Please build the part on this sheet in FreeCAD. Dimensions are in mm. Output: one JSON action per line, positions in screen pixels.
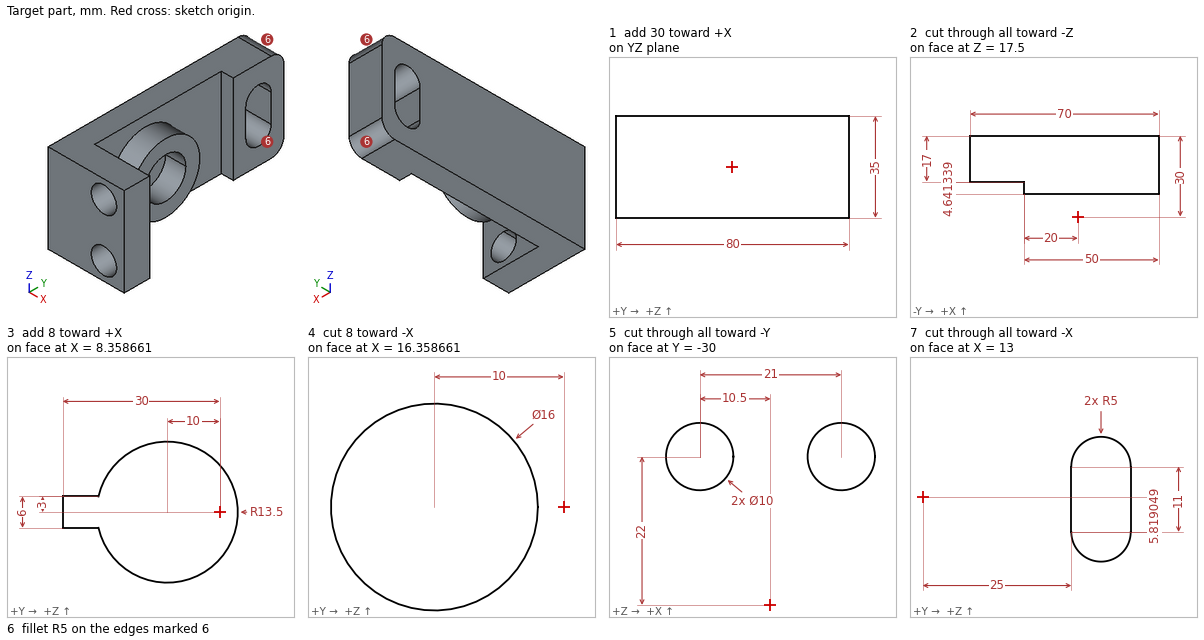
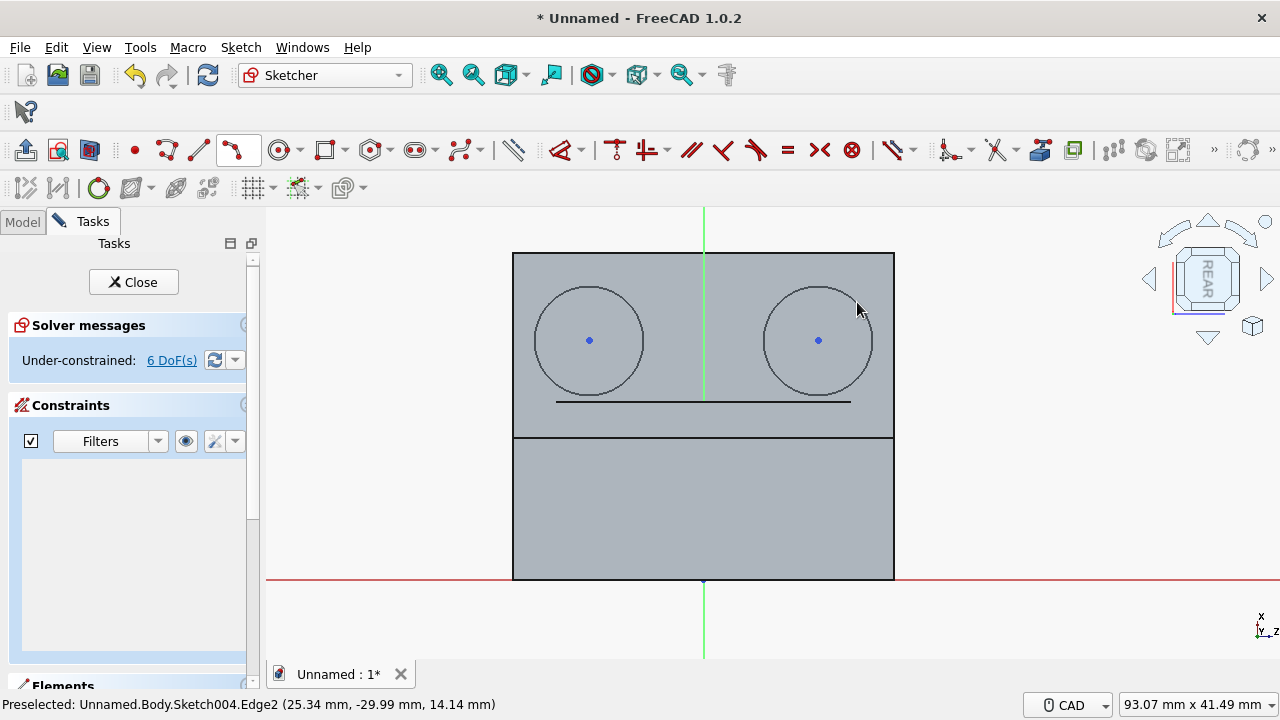
{"action": "left_click", "coordinate": [627, 302]}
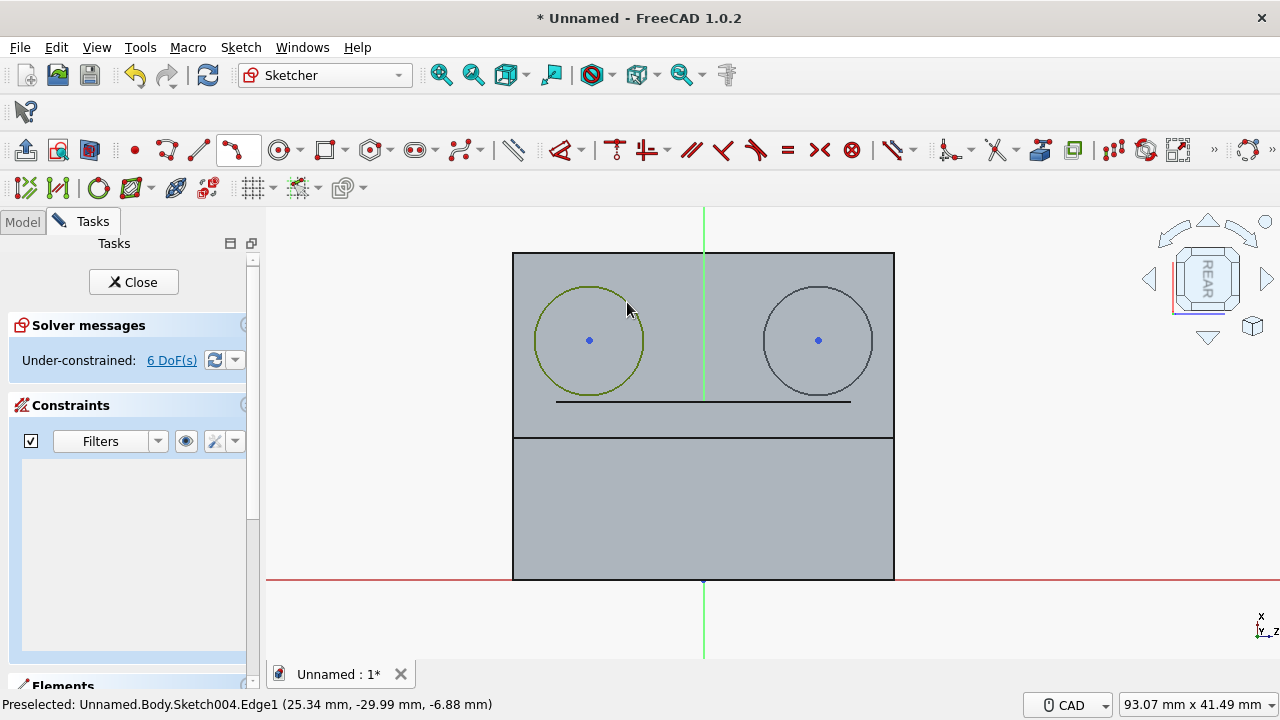
{"action": "left_click", "coordinate": [856, 302]}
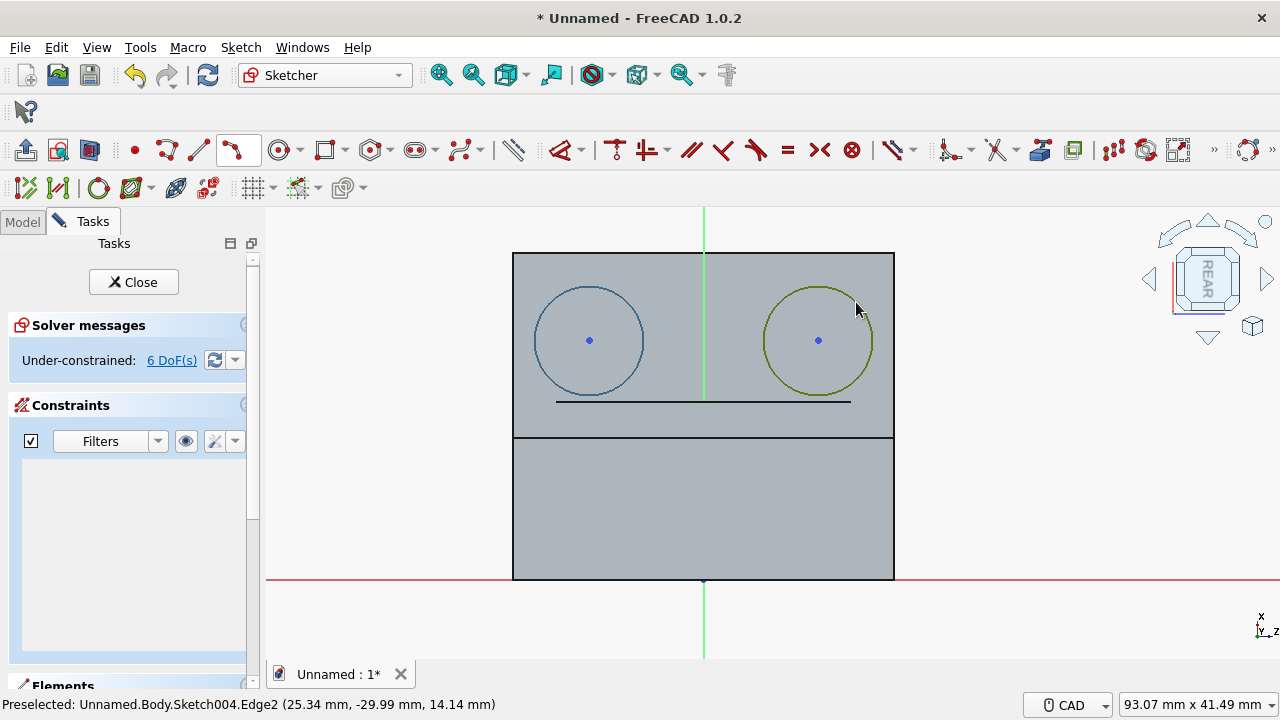
{"action": "left_click", "coordinate": [788, 150]}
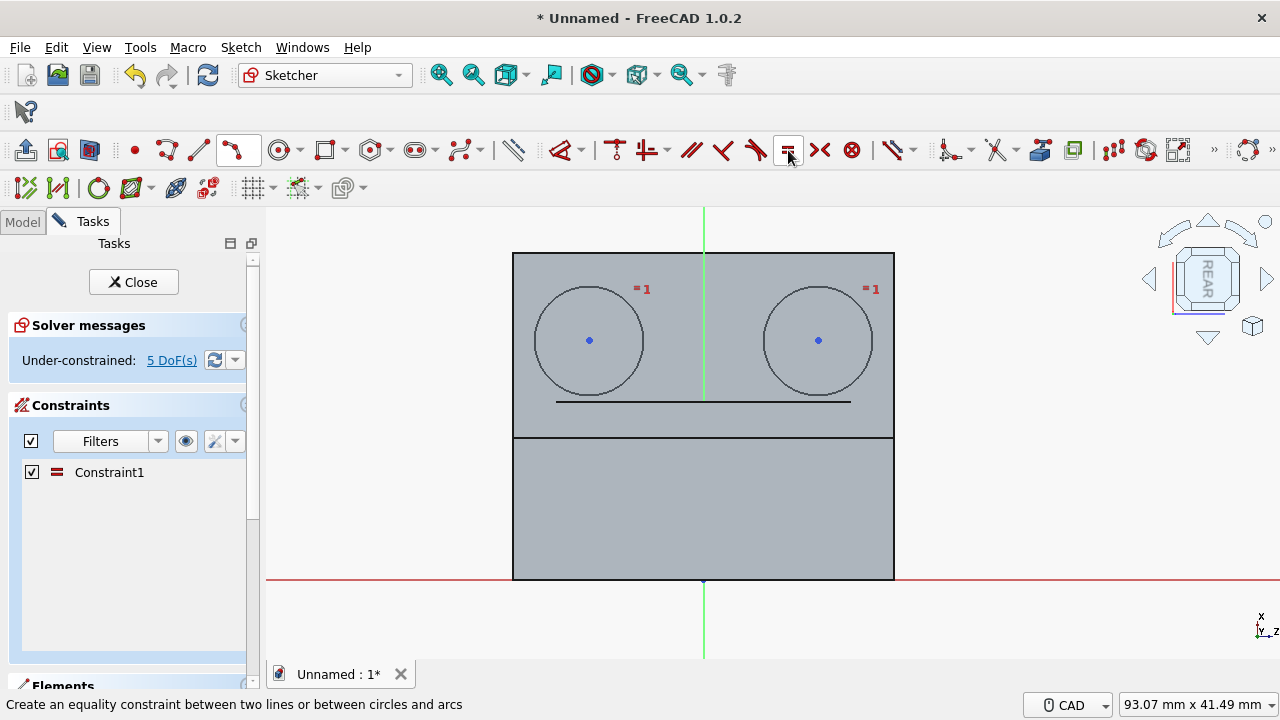
{"action": "left_click", "coordinate": [589, 341]}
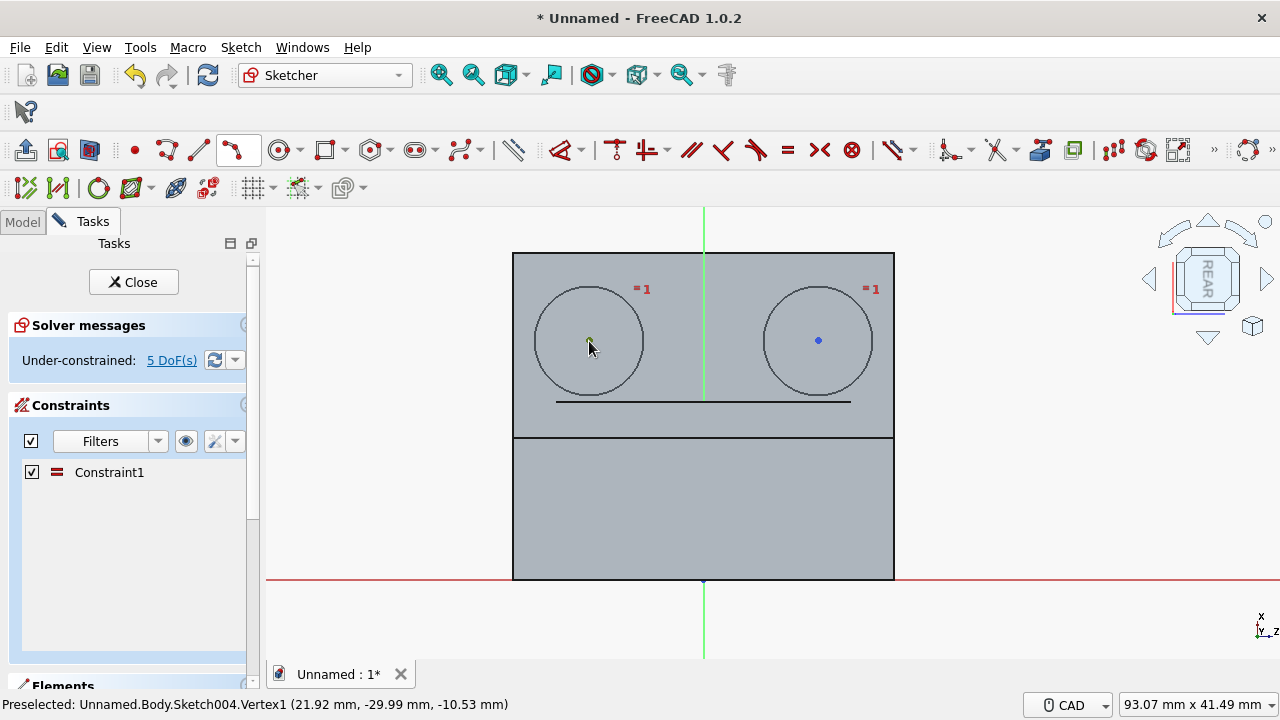
{"action": "left_click", "coordinate": [818, 341]}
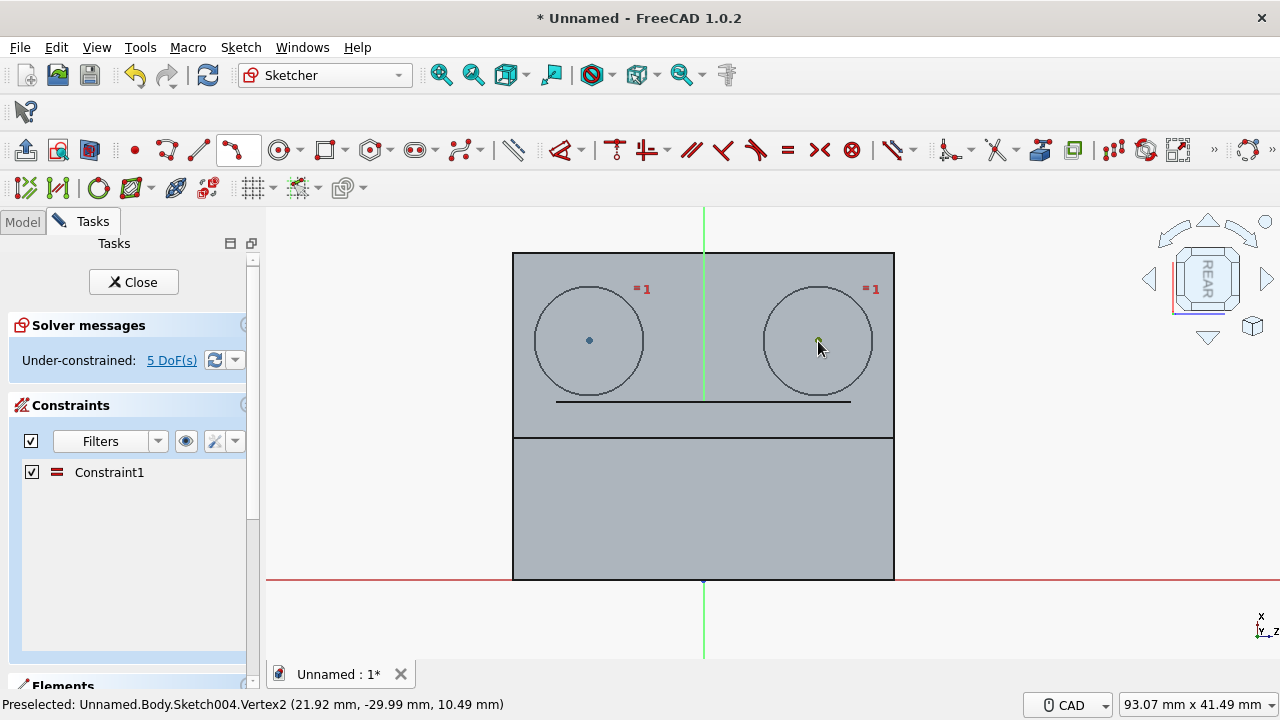
{"action": "left_click", "coordinate": [670, 150]}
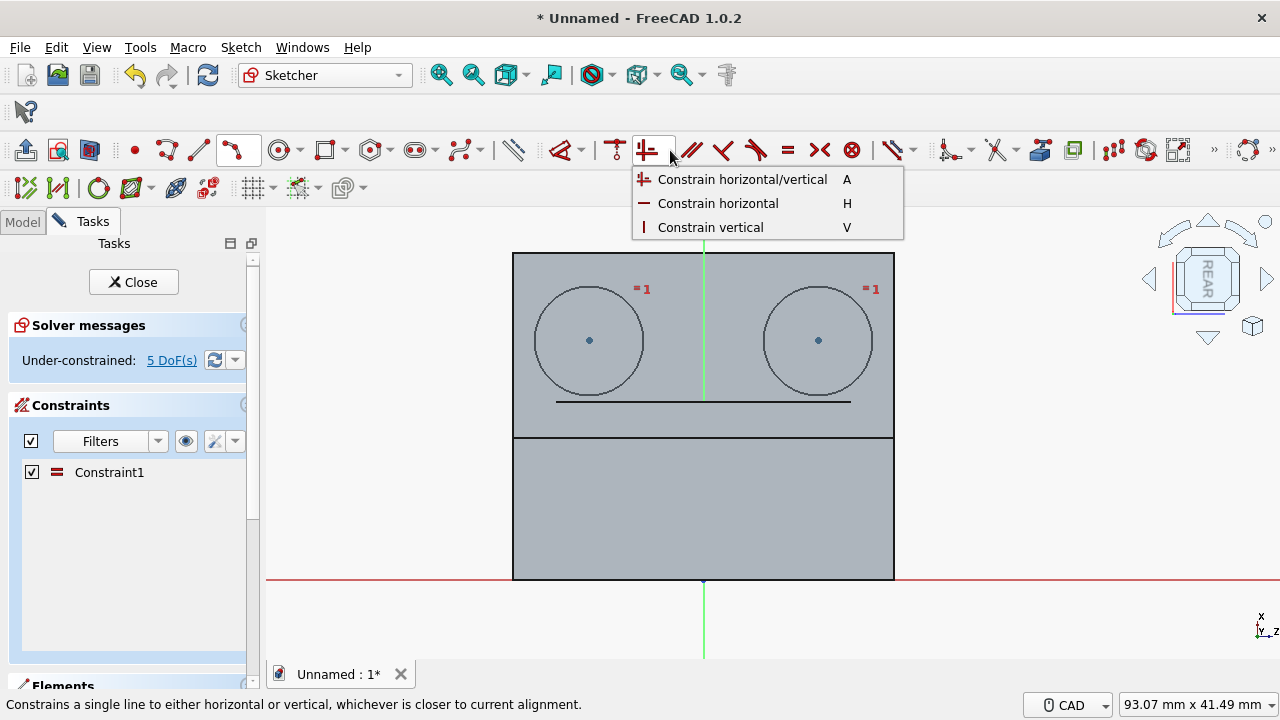
{"action": "left_click", "coordinate": [768, 203]}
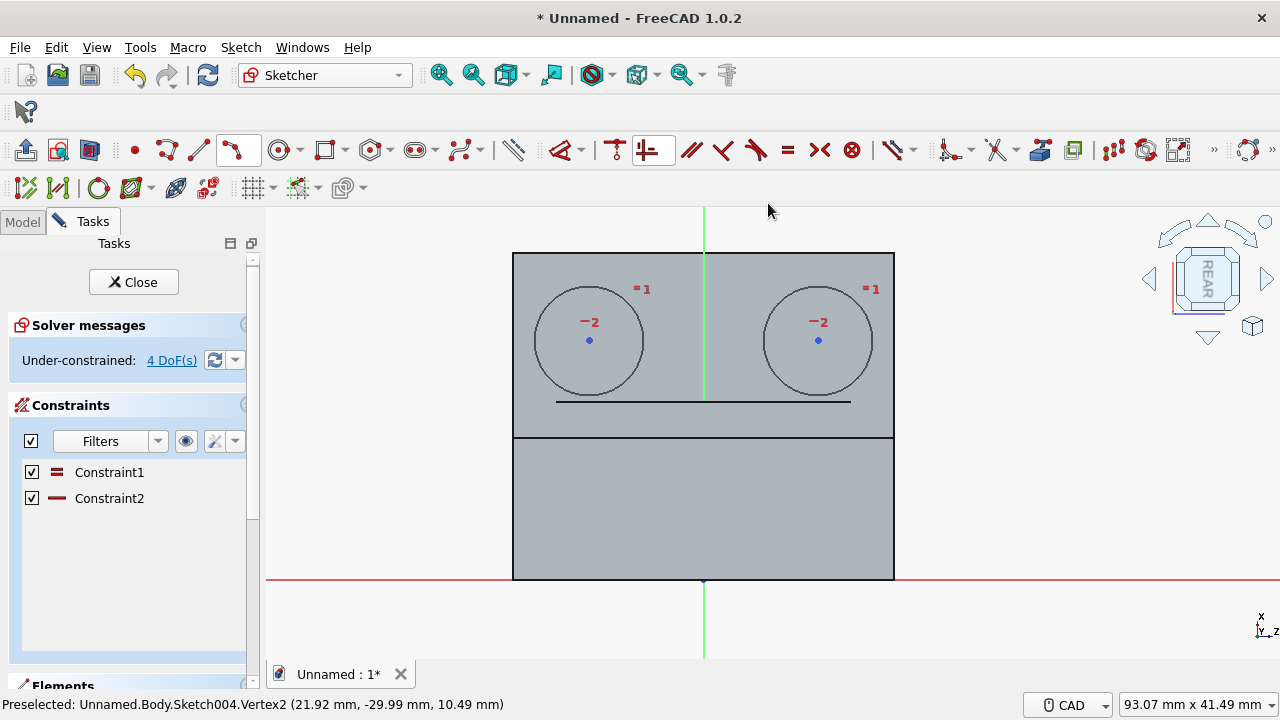
{"action": "left_click", "coordinate": [560, 150]}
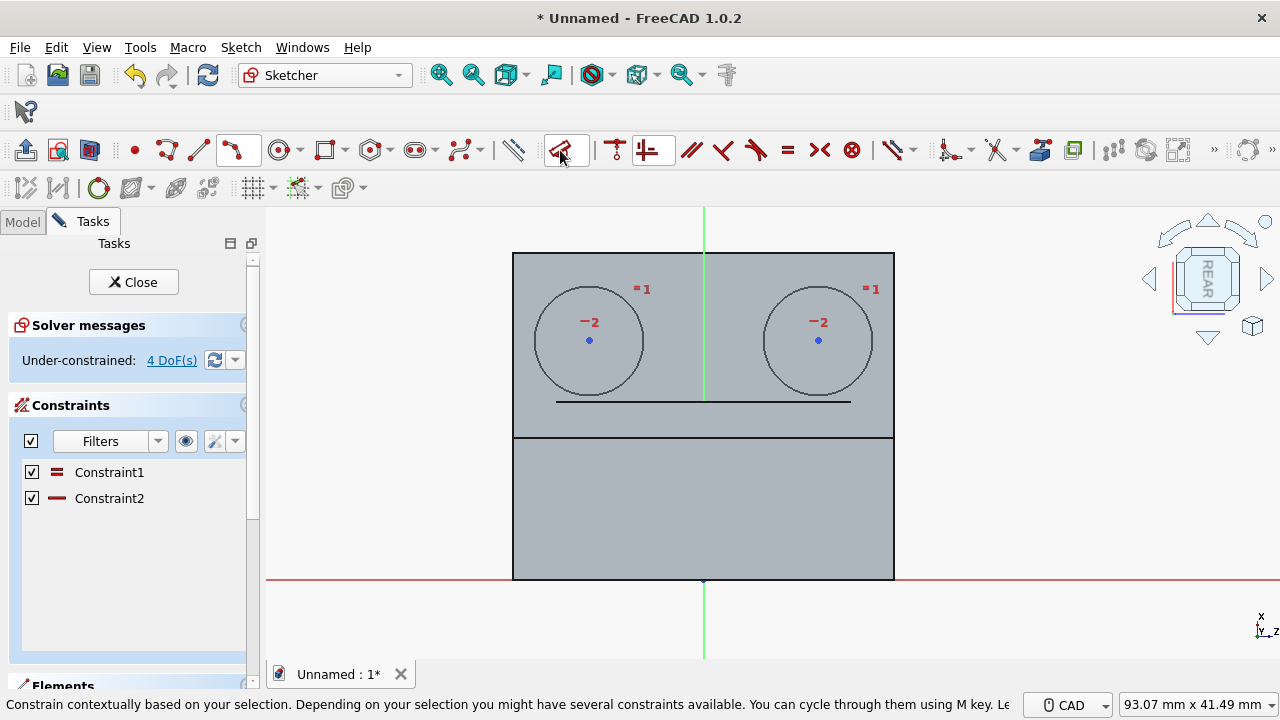
{"action": "left_click", "coordinate": [627, 302]}
{"action": "left_click", "coordinate": [649, 279]}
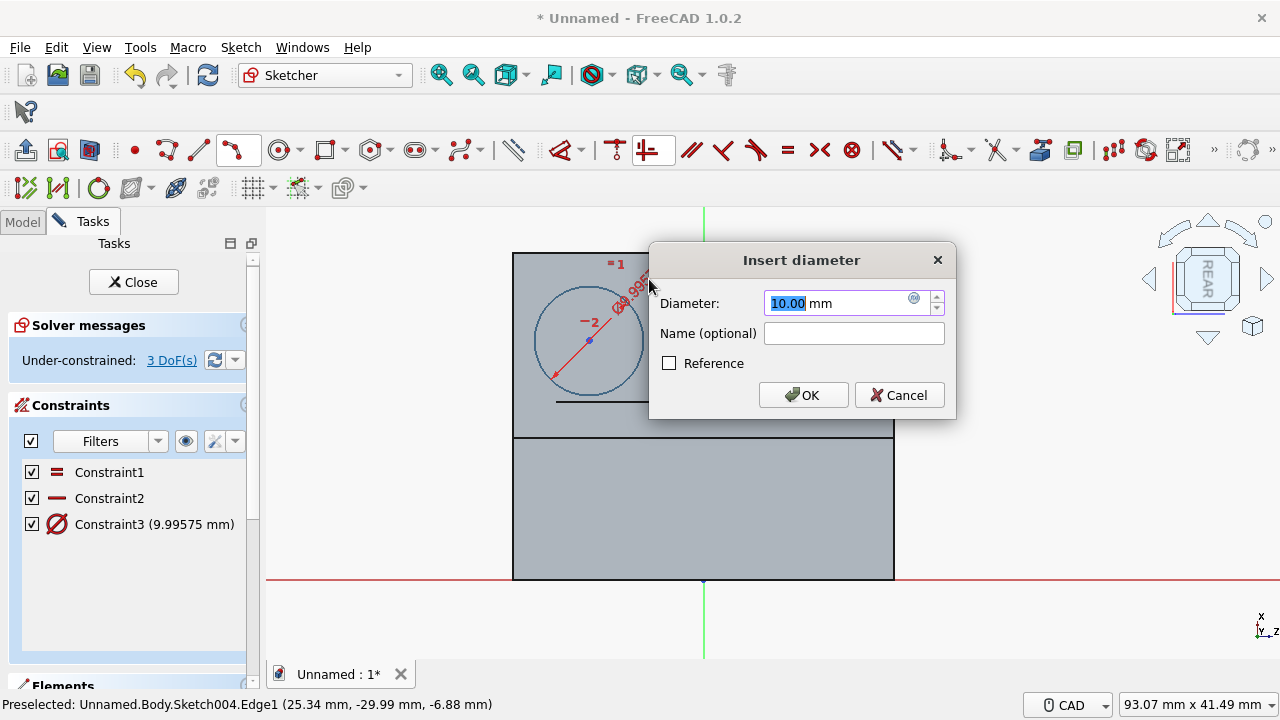
{"action": "type", "text": "10"}
{"action": "key", "text": "Return"}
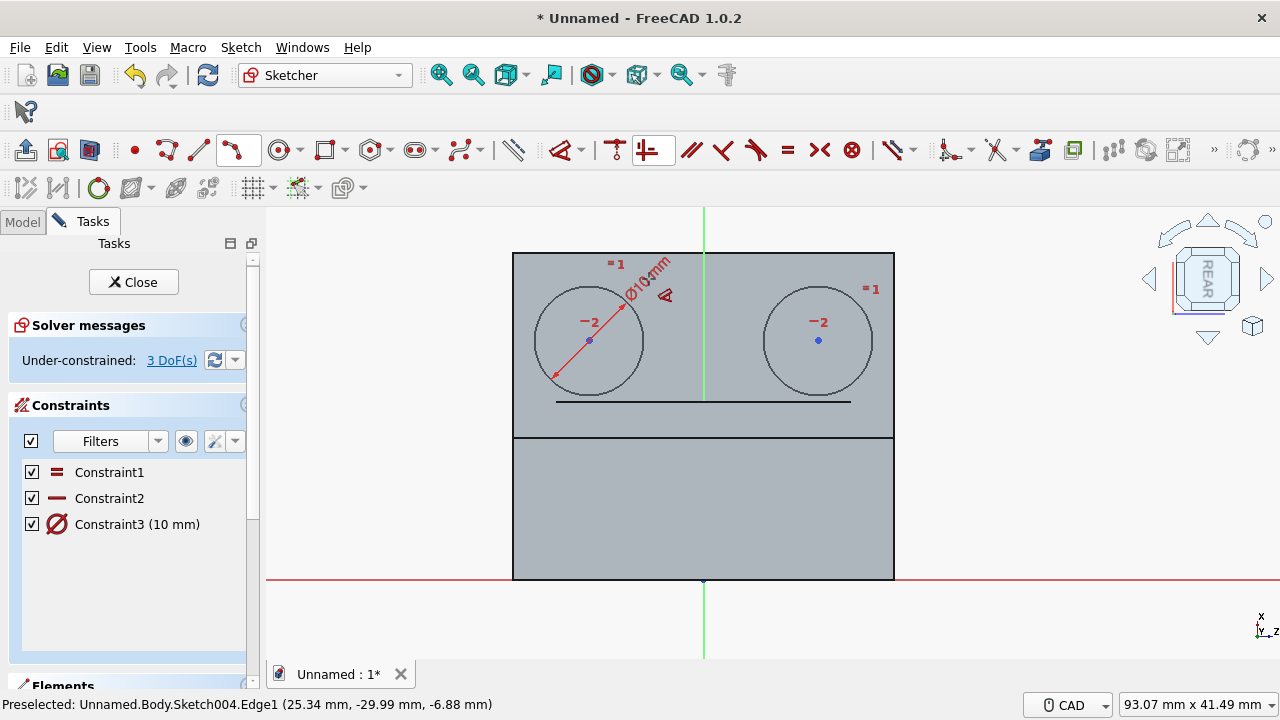
{"action": "left_click", "coordinate": [589, 341]}
{"action": "left_click", "coordinate": [555, 460]}